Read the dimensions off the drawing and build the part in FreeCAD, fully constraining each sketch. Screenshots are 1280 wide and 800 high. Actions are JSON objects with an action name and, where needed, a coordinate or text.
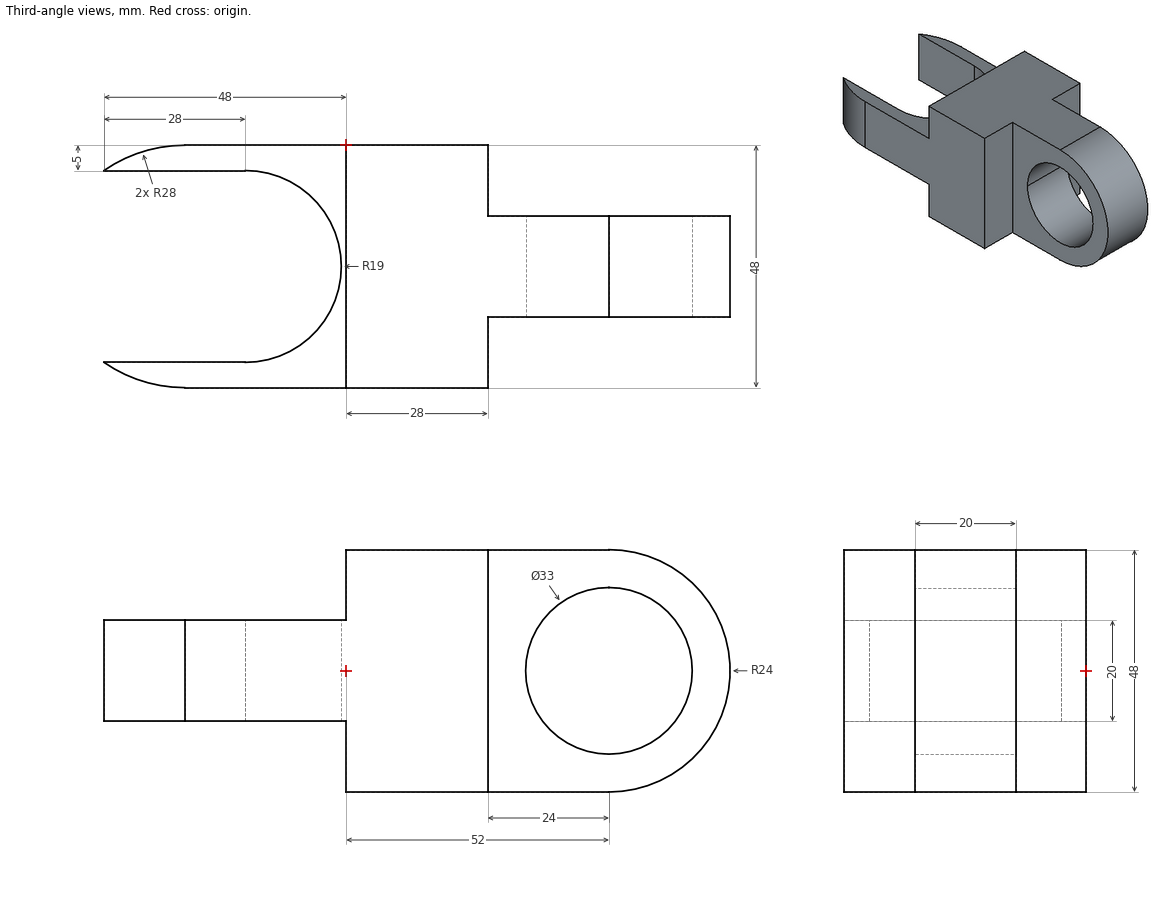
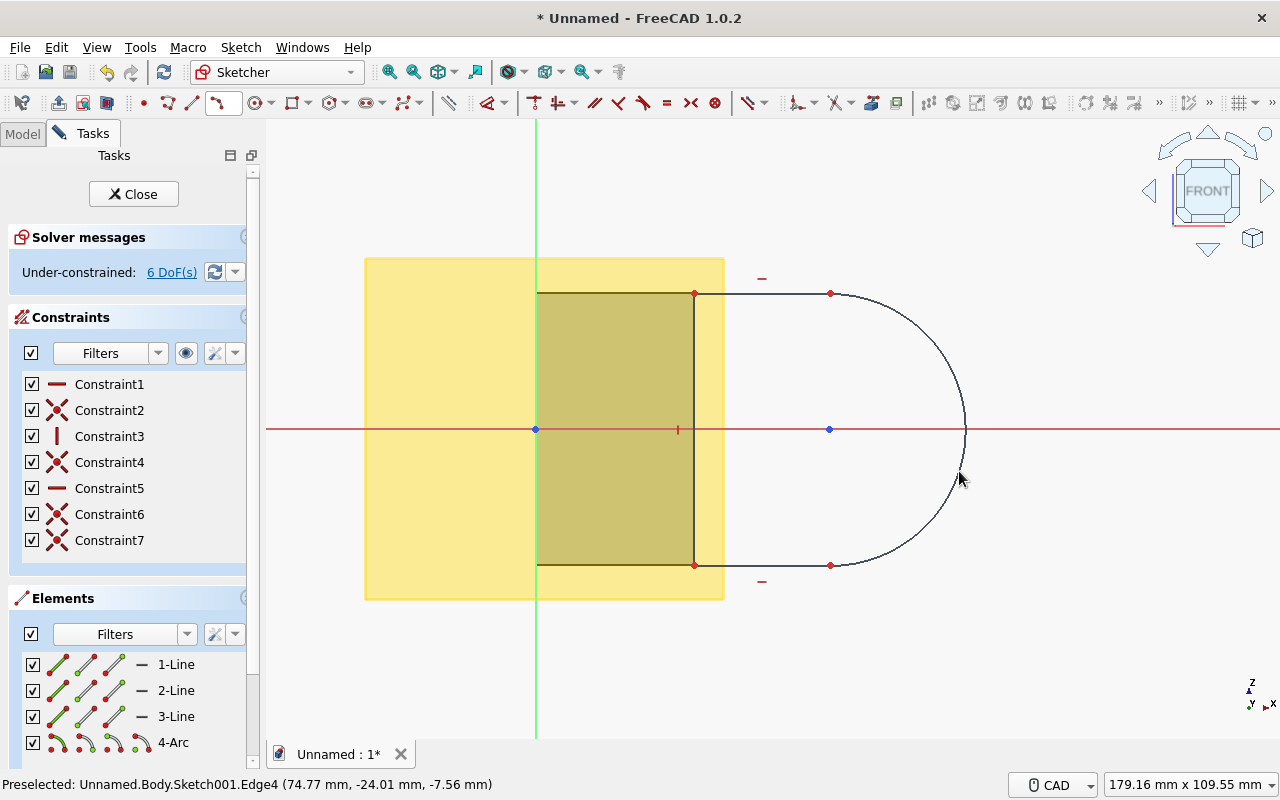
{"action": "left_click", "coordinate": [789, 566]}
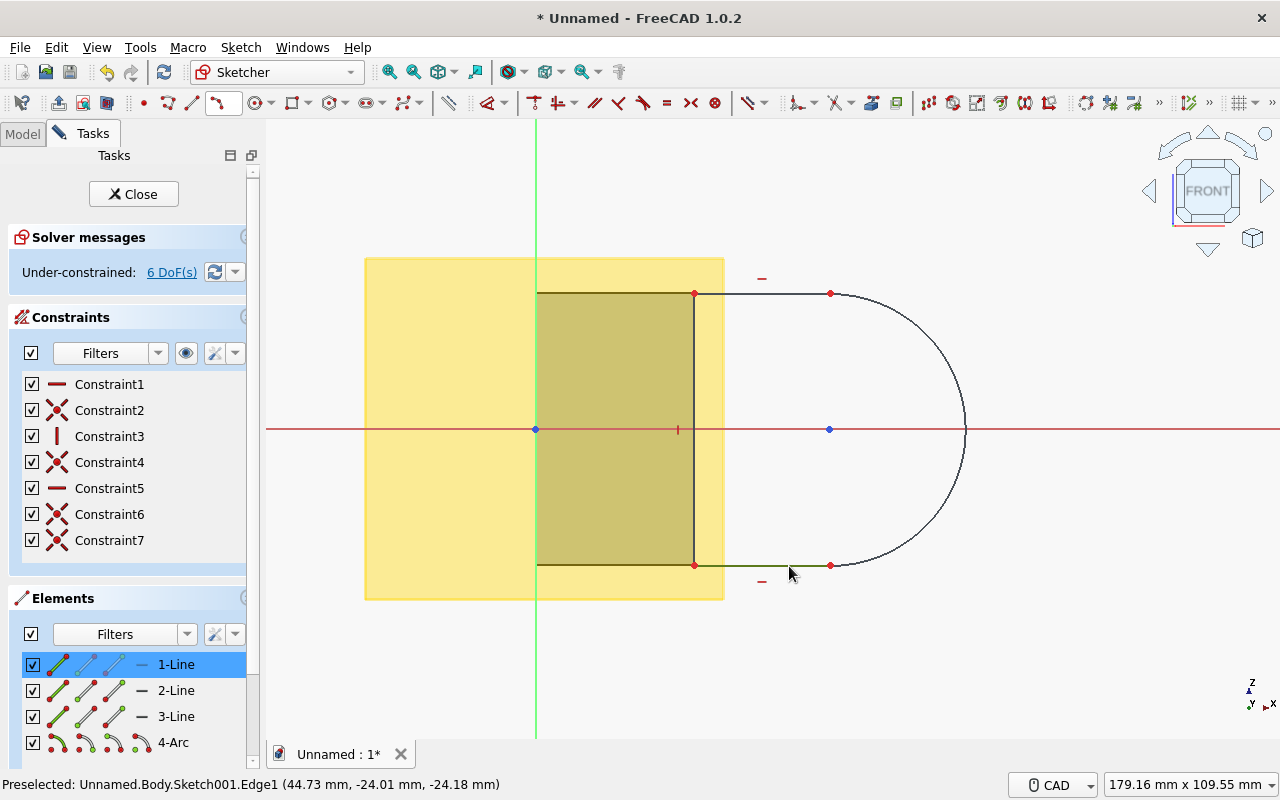
{"action": "left_click", "coordinate": [940, 510]}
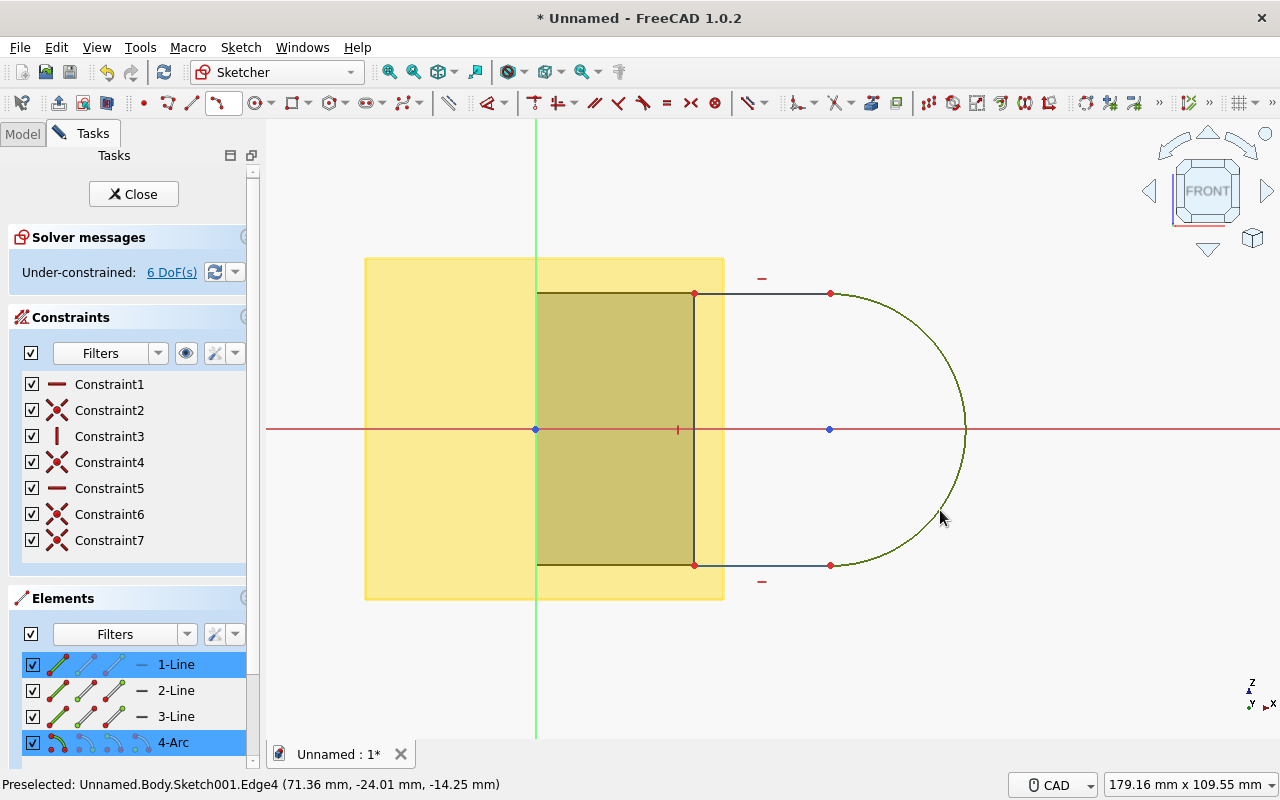
{"action": "left_click", "coordinate": [644, 104]}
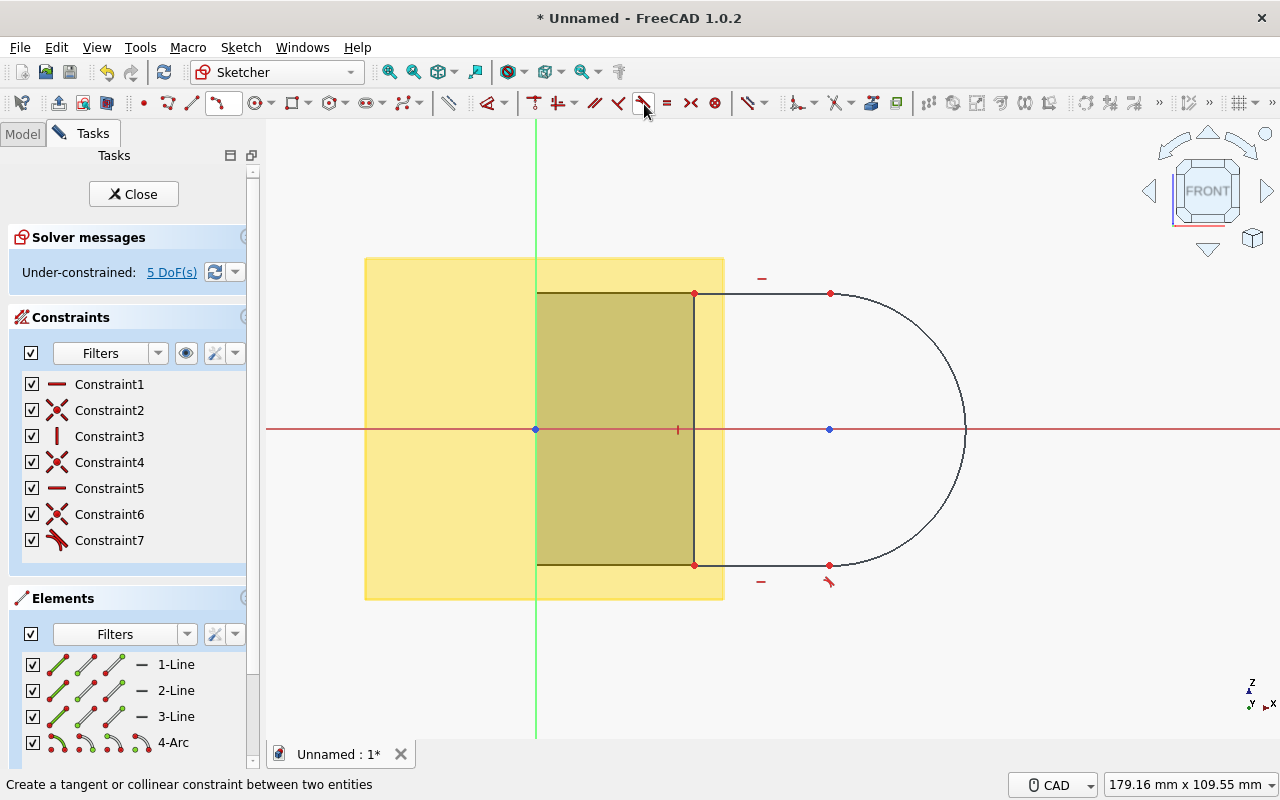
{"action": "left_click", "coordinate": [735, 294]}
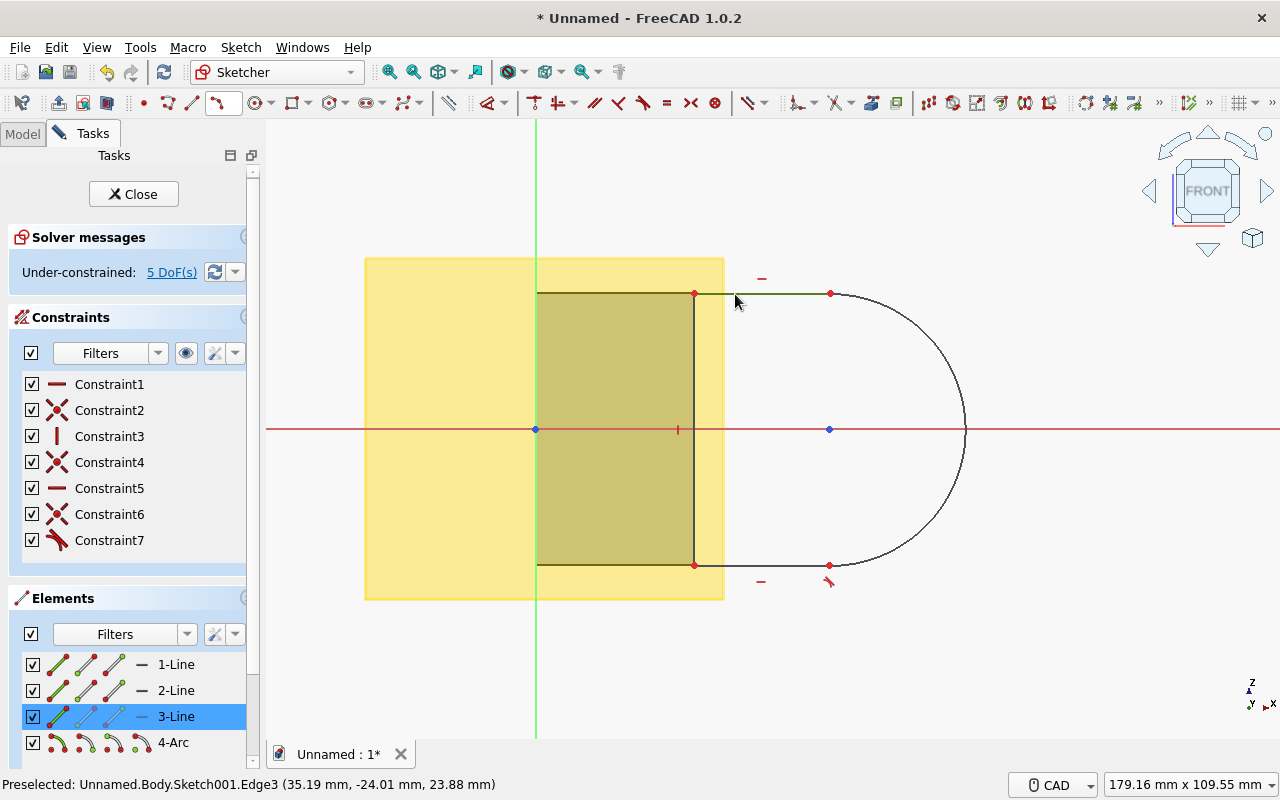
{"action": "left_click", "coordinate": [940, 510]}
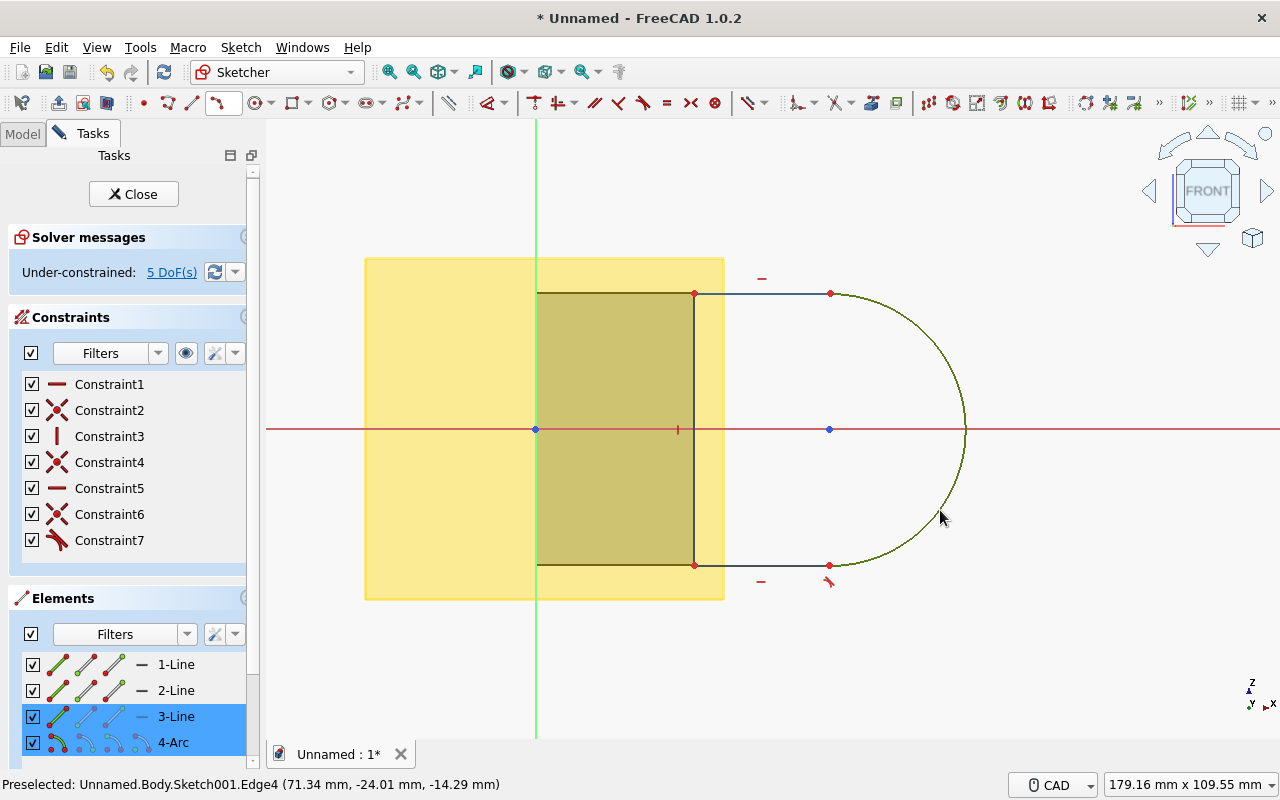
{"action": "left_click", "coordinate": [644, 104]}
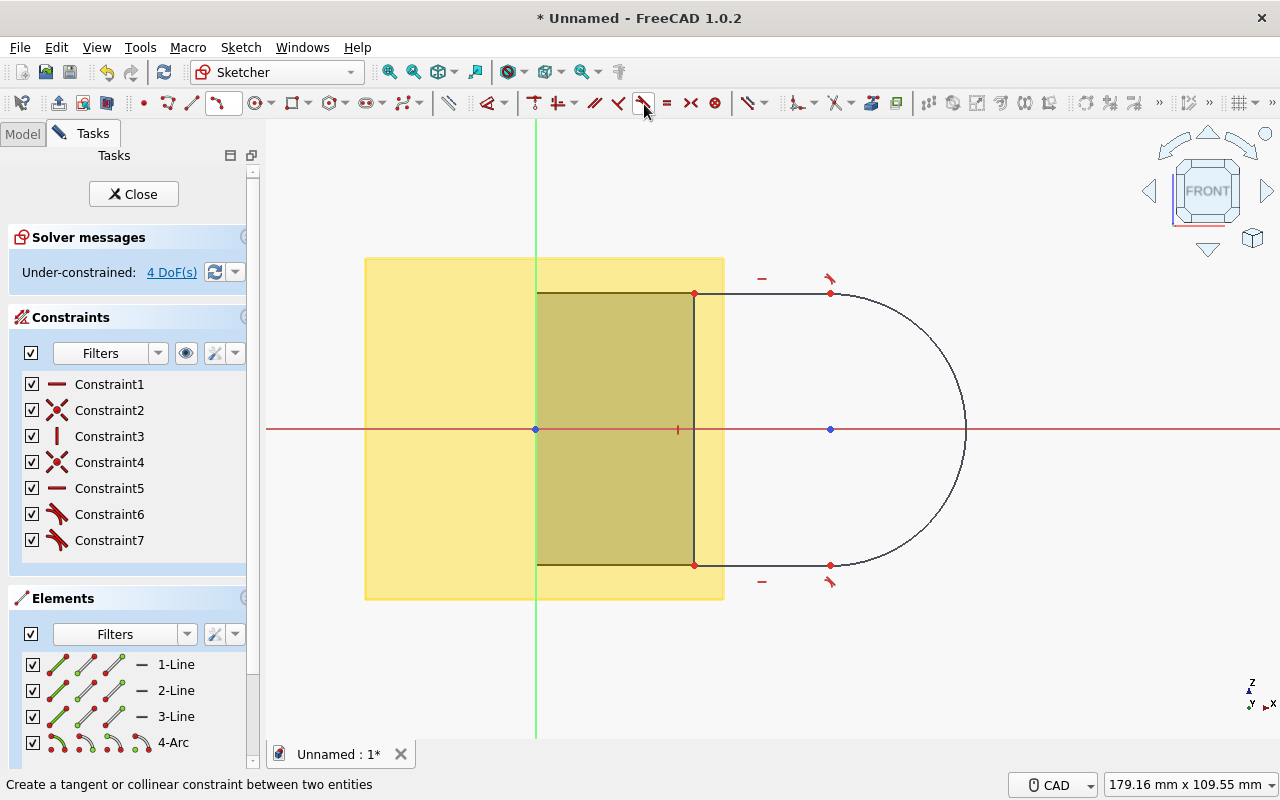
{"action": "left_click", "coordinate": [830, 430]}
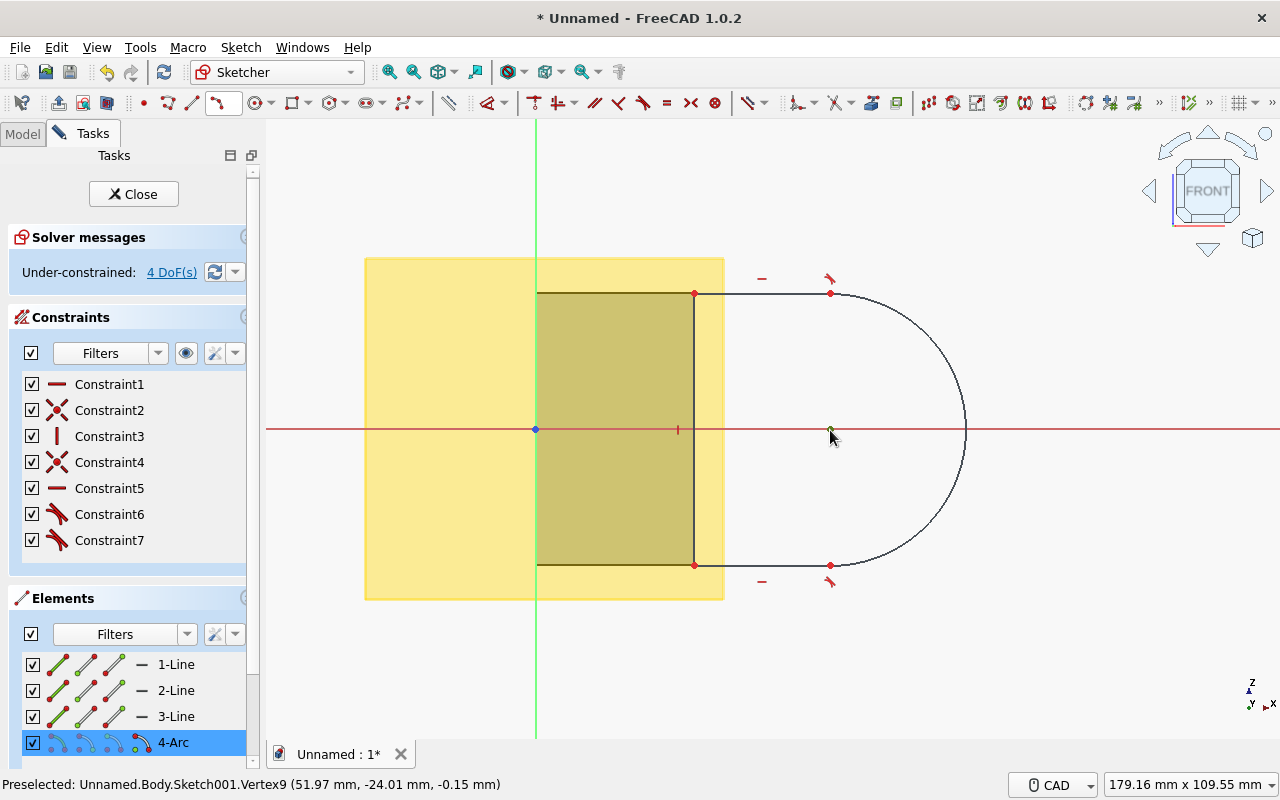
{"action": "left_click", "coordinate": [353, 429]}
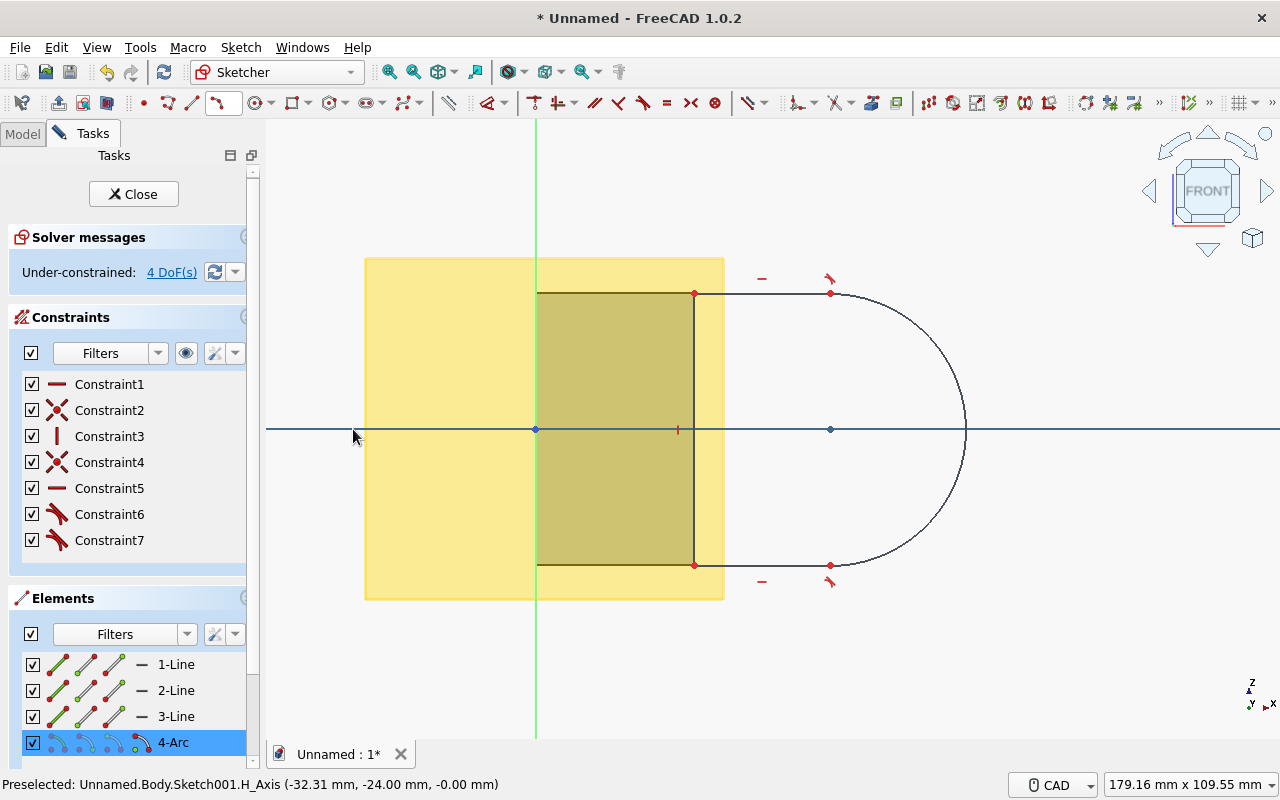
{"action": "left_click", "coordinate": [534, 104]}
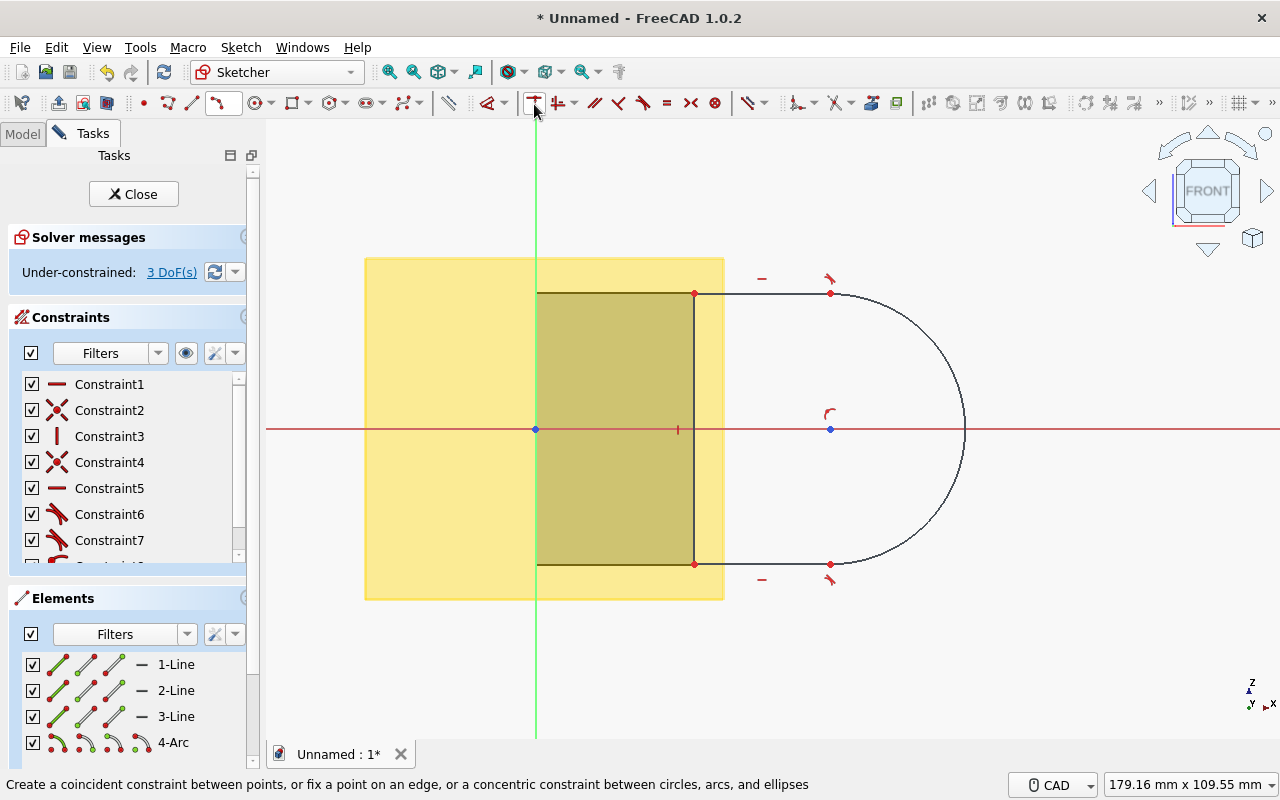
{"action": "left_click", "coordinate": [488, 104]}